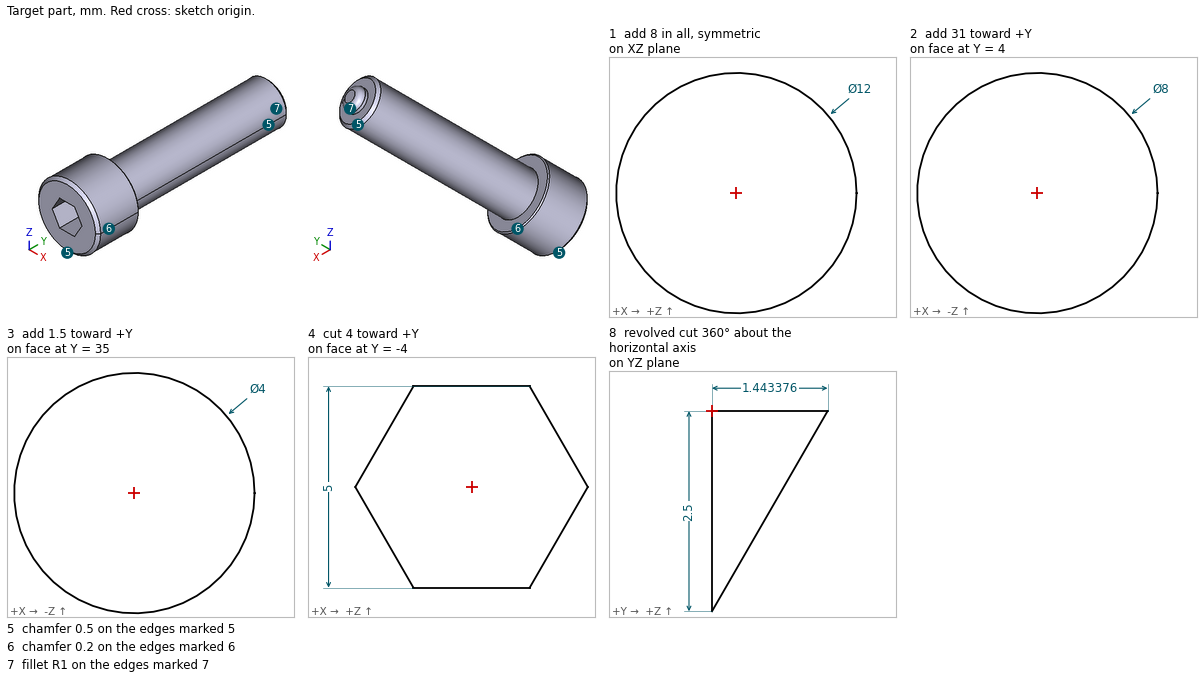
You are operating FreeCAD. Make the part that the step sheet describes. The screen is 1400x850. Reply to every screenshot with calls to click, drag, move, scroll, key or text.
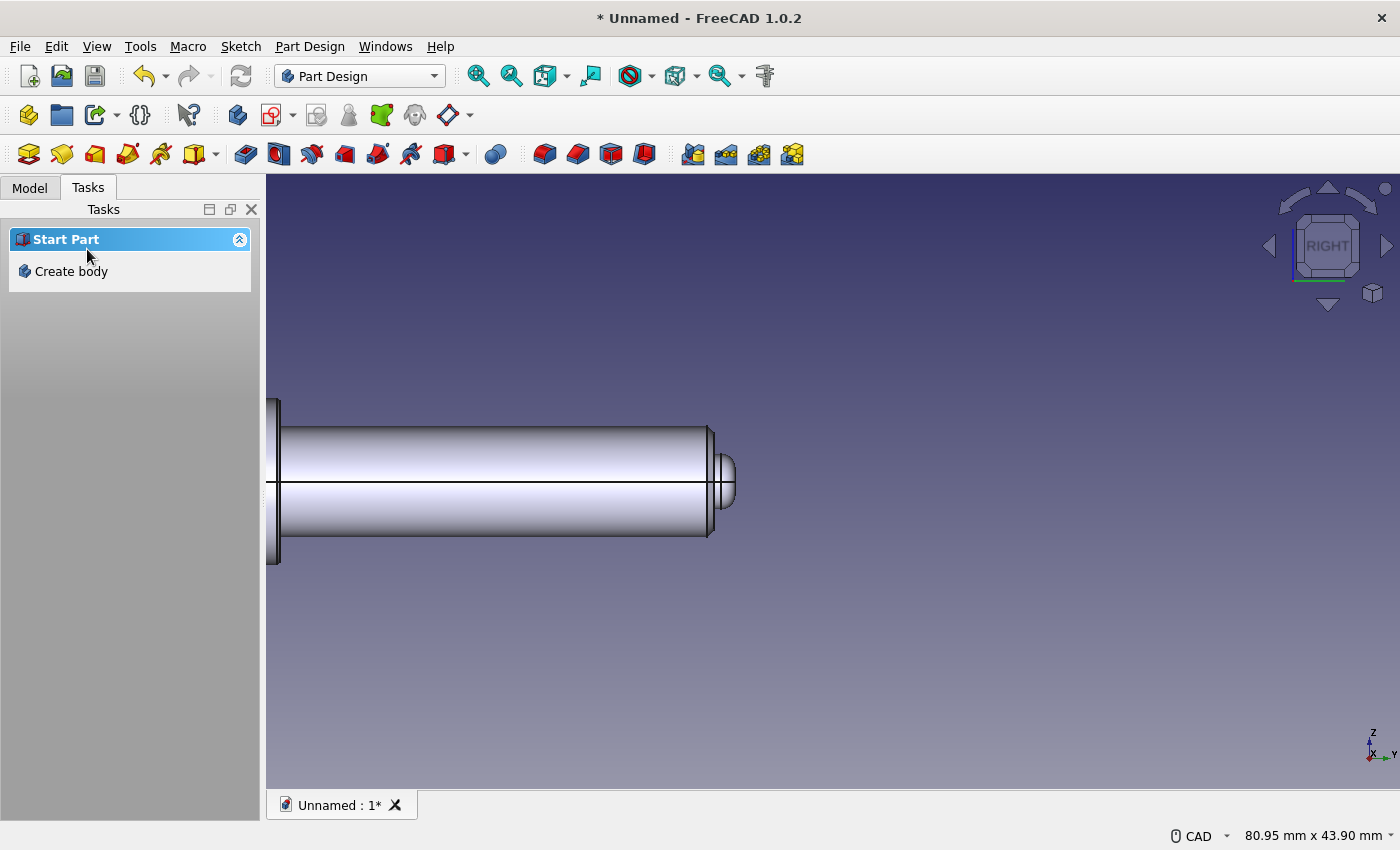
key(0)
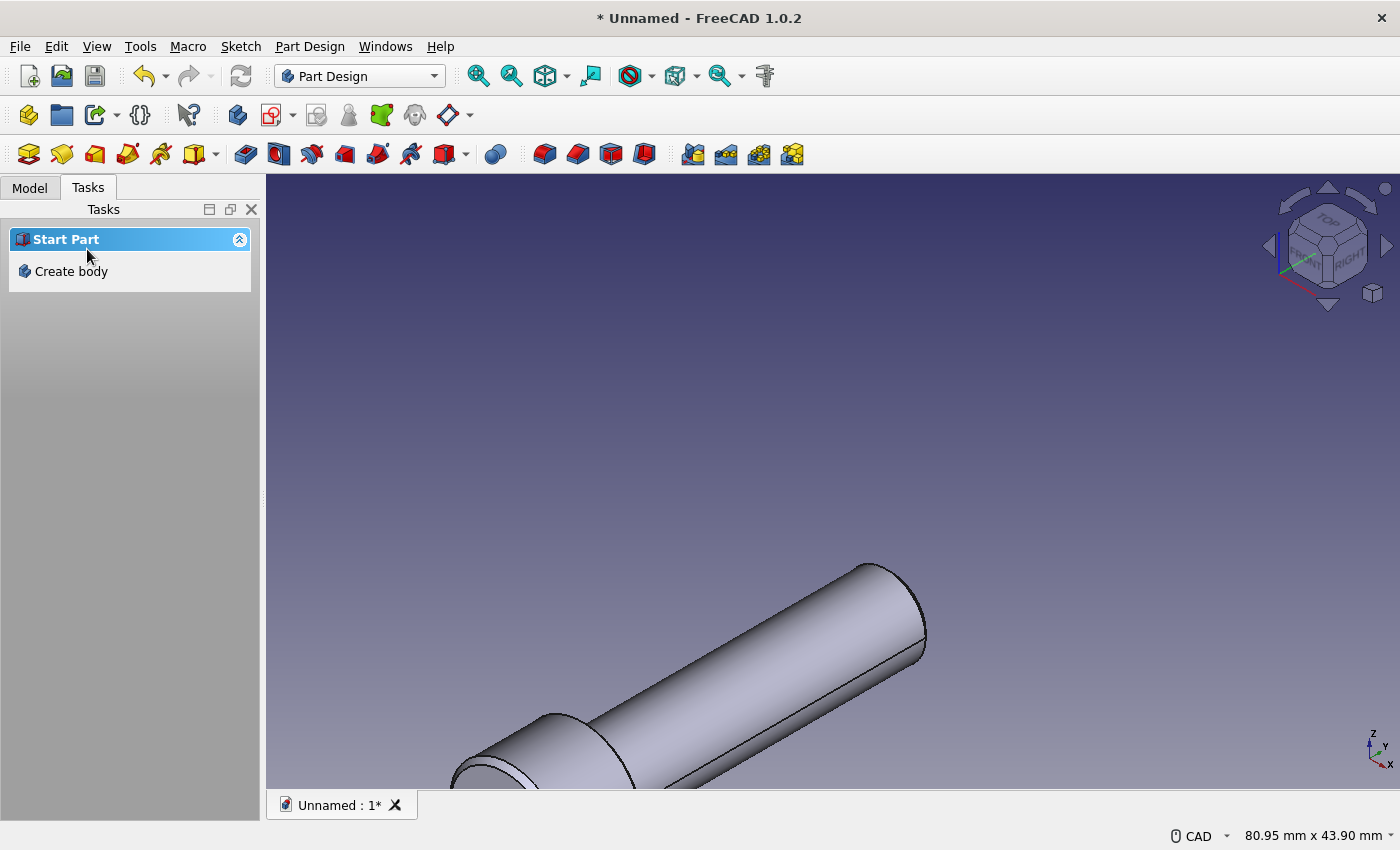
click(479, 76)